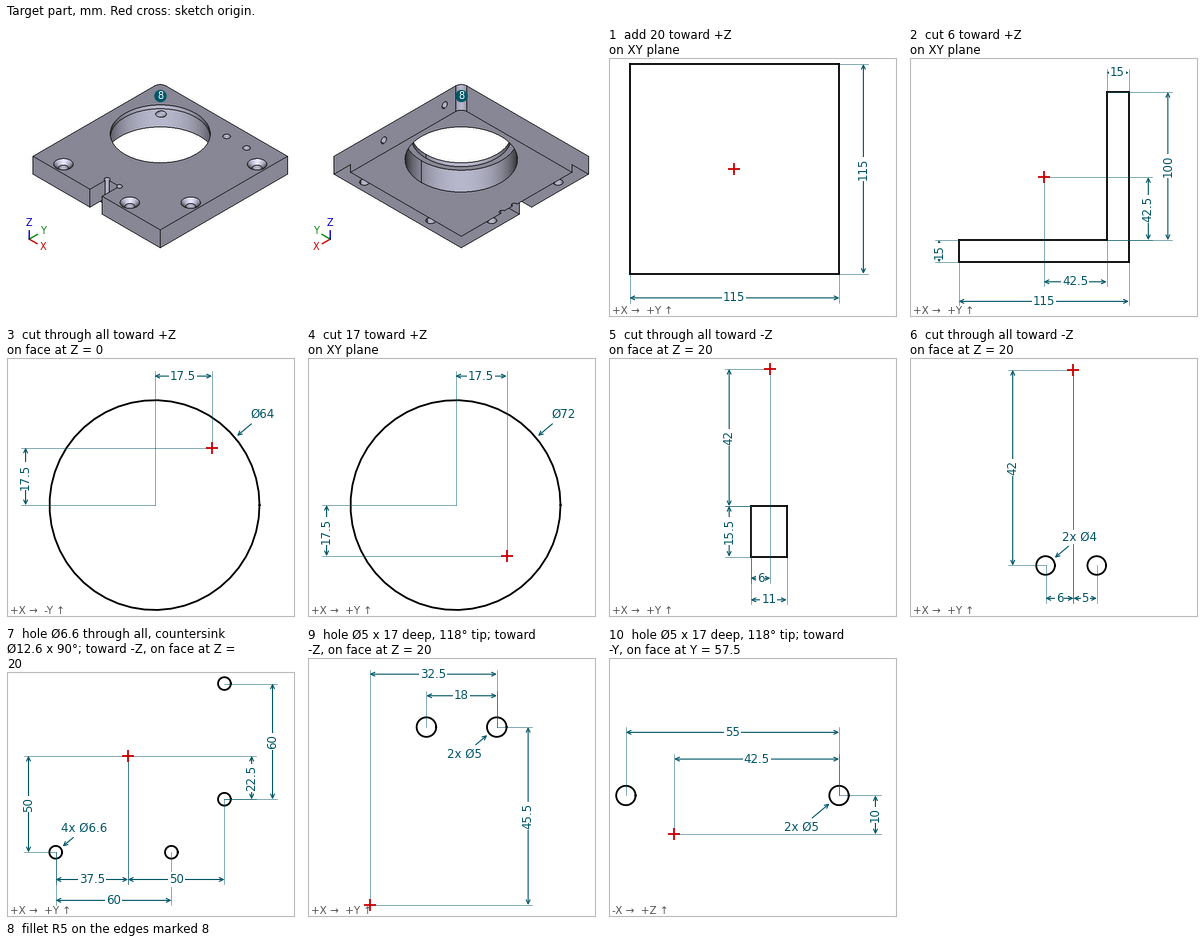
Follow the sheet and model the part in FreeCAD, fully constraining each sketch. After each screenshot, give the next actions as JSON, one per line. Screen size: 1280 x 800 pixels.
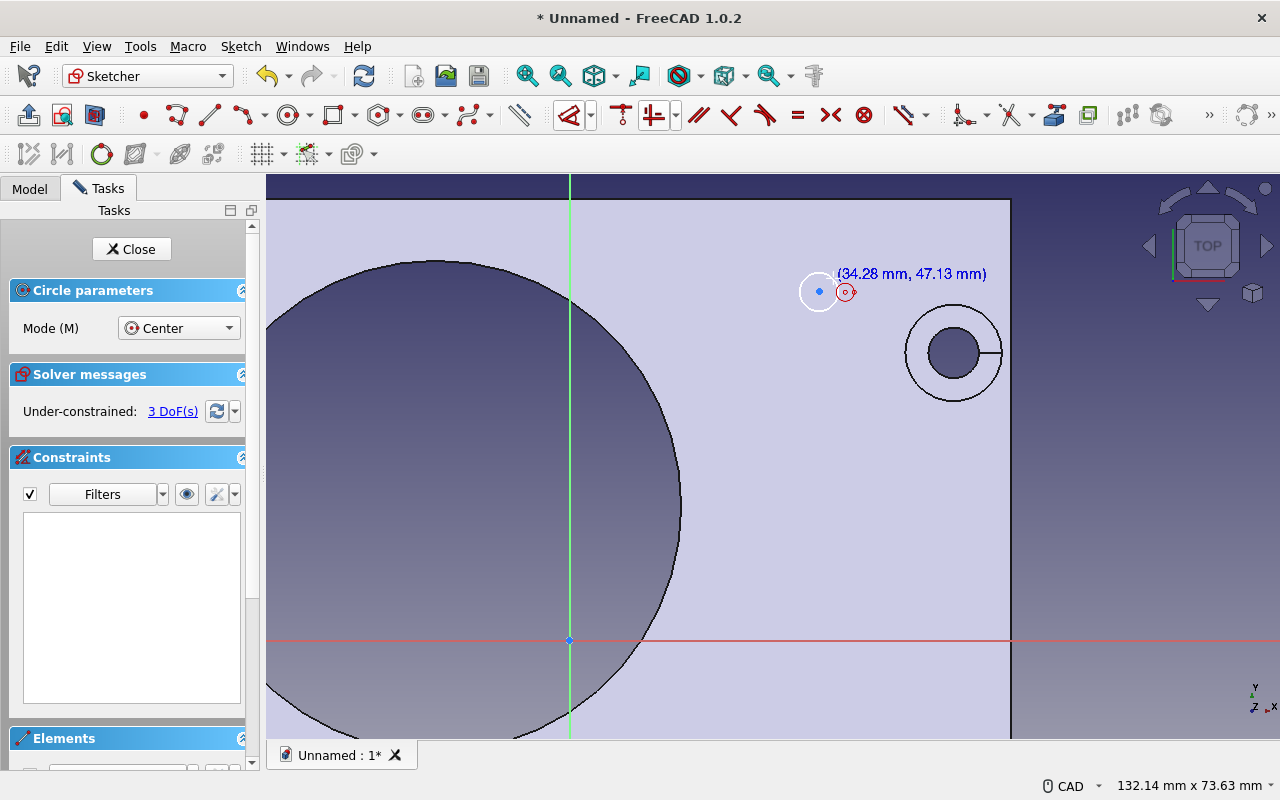
{"action": "left_click", "coordinate": [681, 291]}
{"action": "left_click", "coordinate": [695, 278]}
{"action": "key", "text": "Escape"}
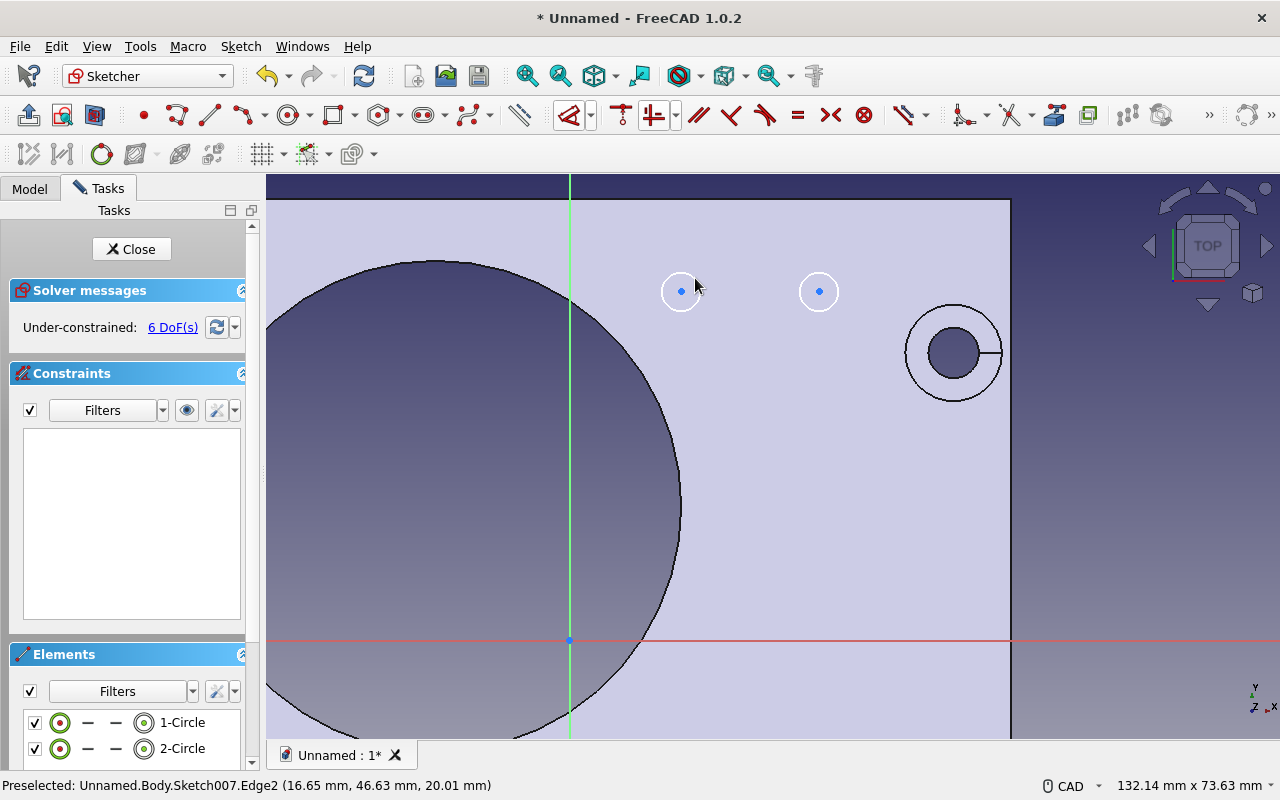
{"action": "left_click", "coordinate": [832, 278]}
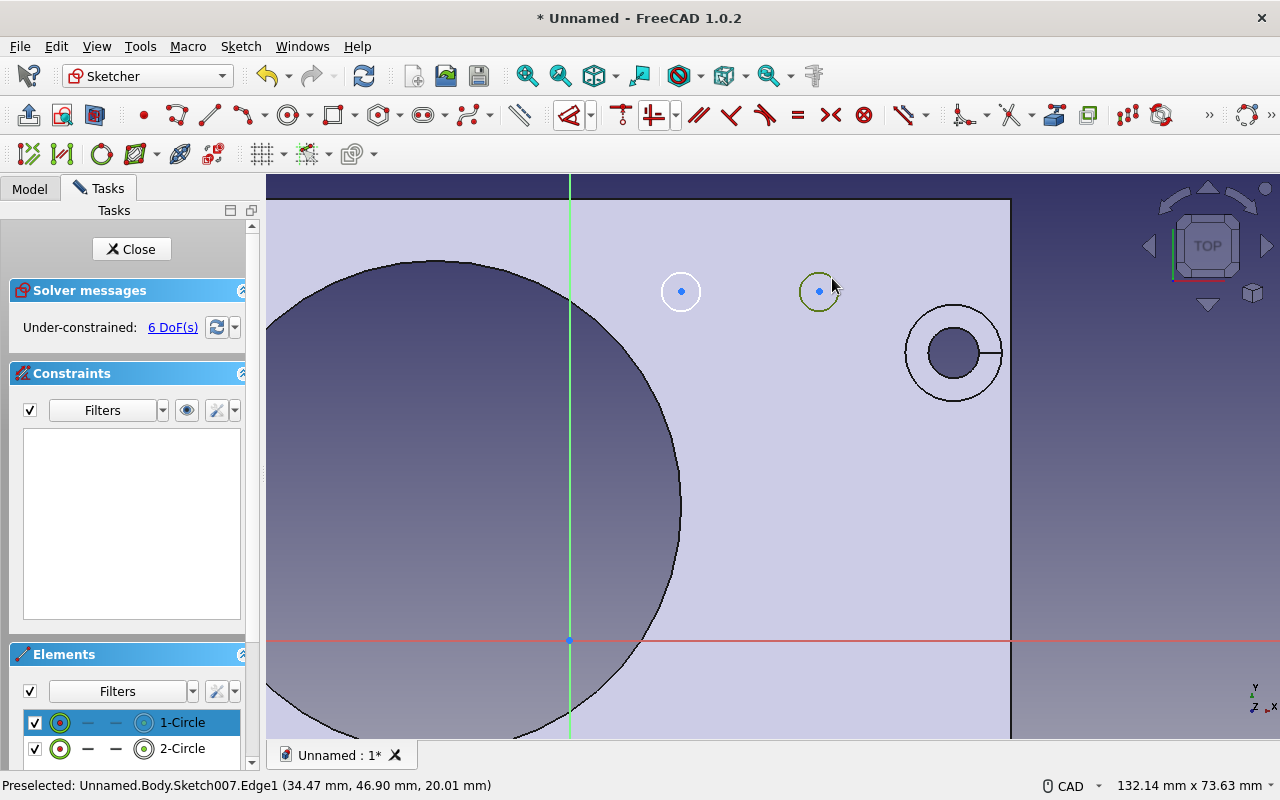
{"action": "left_click", "coordinate": [694, 278]}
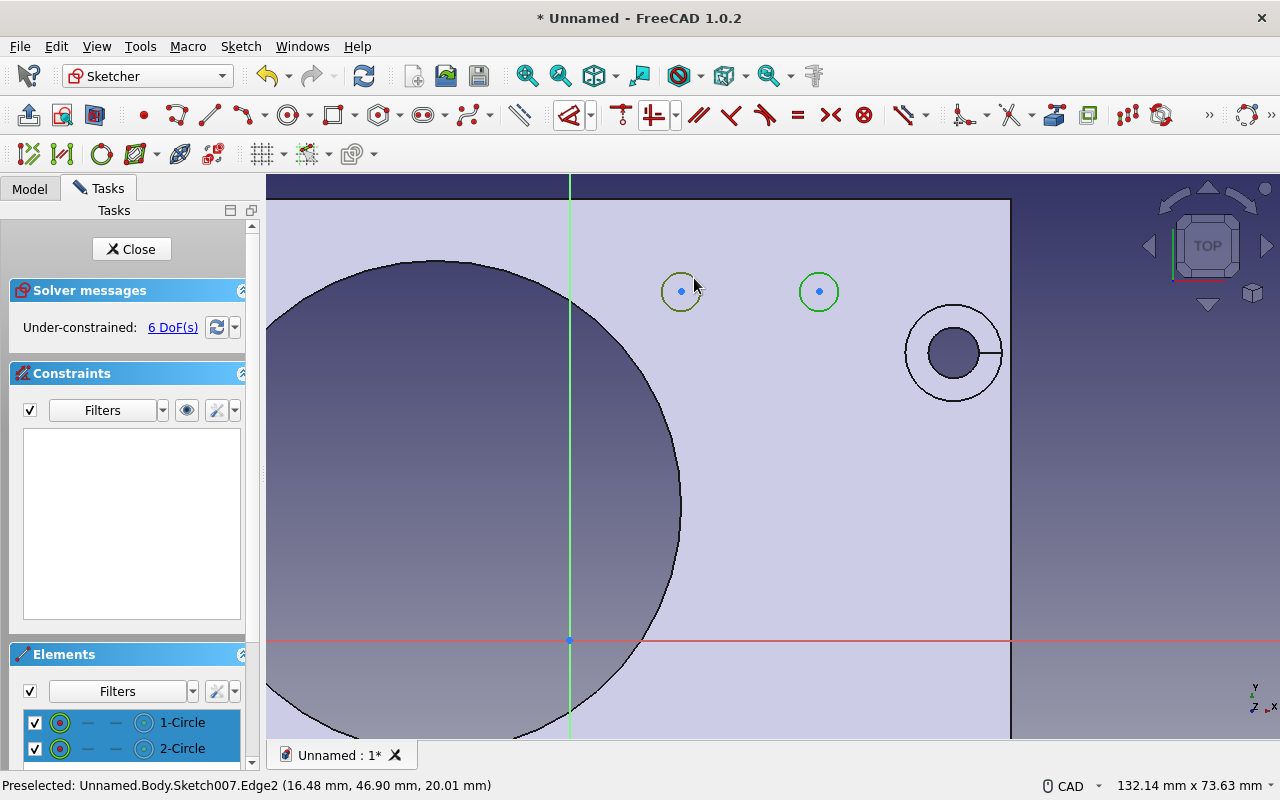
{"action": "left_click", "coordinate": [798, 116]}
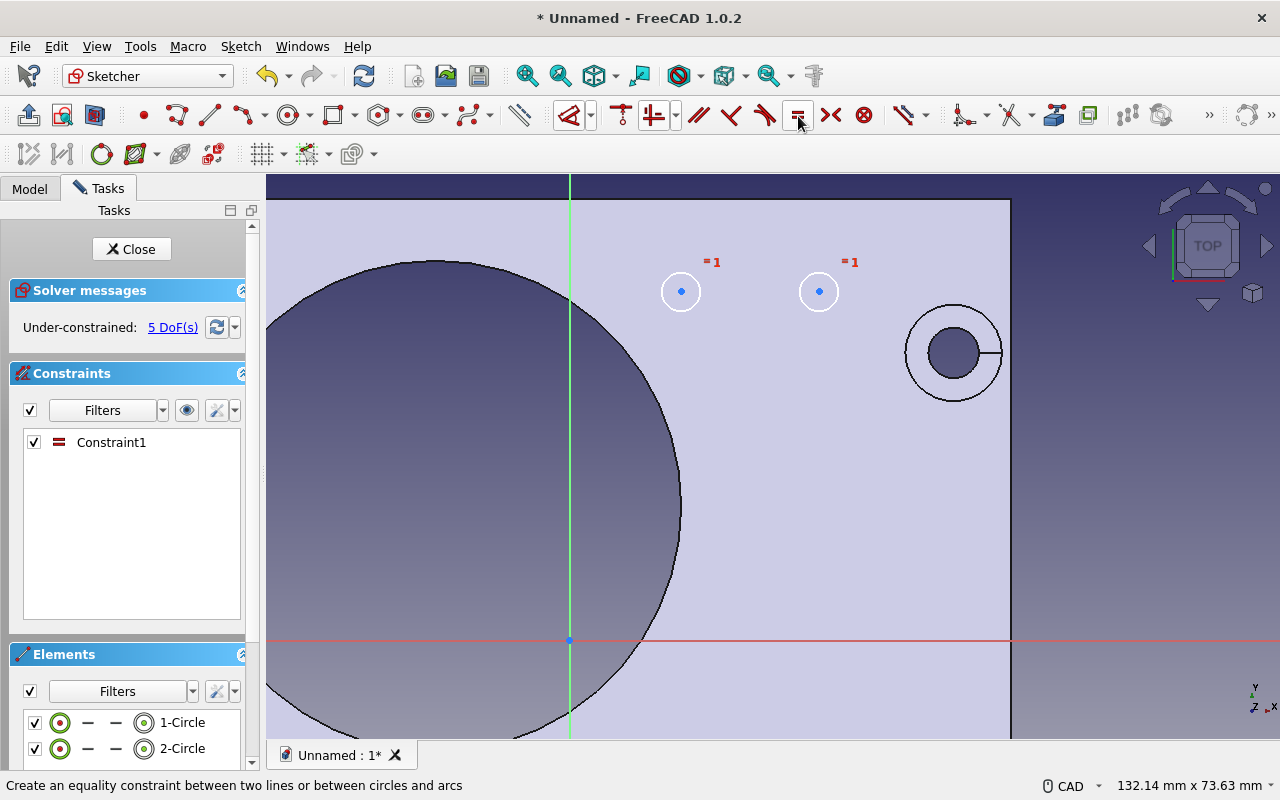
{"action": "left_click", "coordinate": [819, 292]}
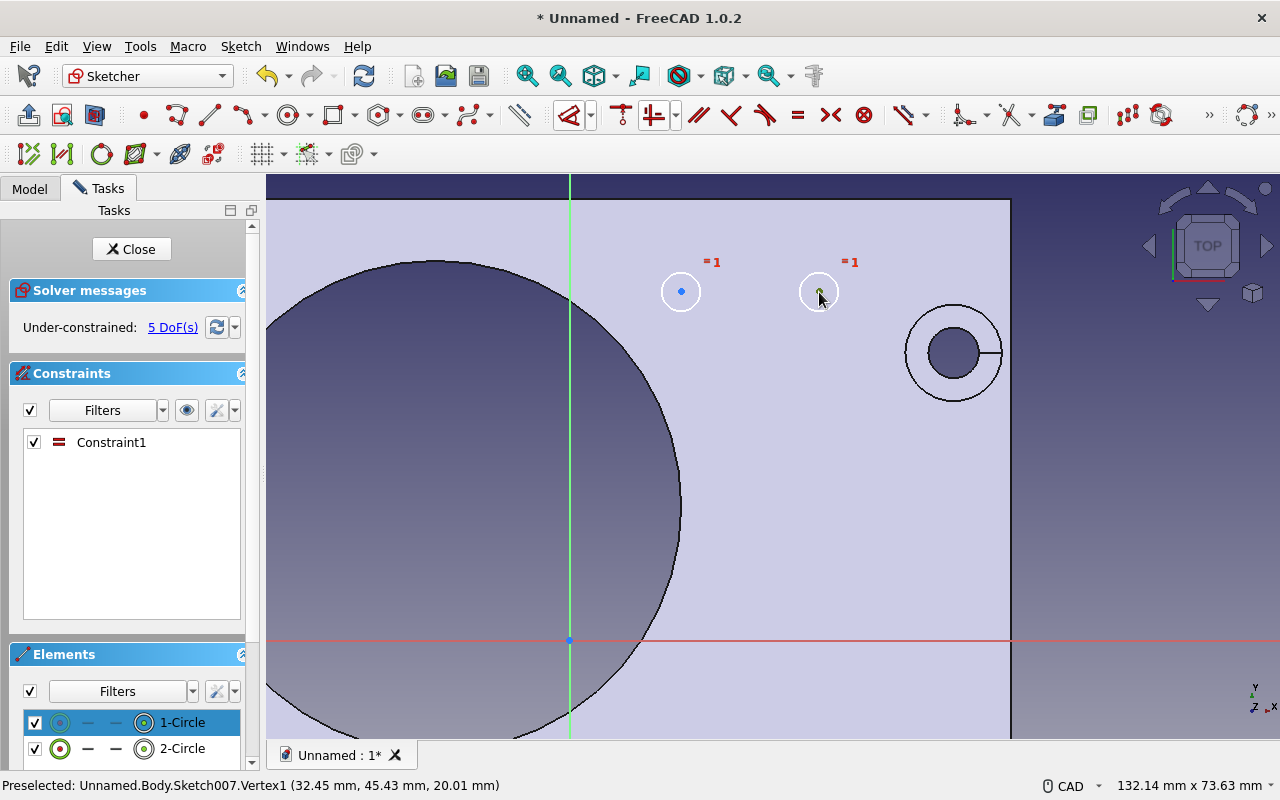
{"action": "left_click", "coordinate": [681, 292]}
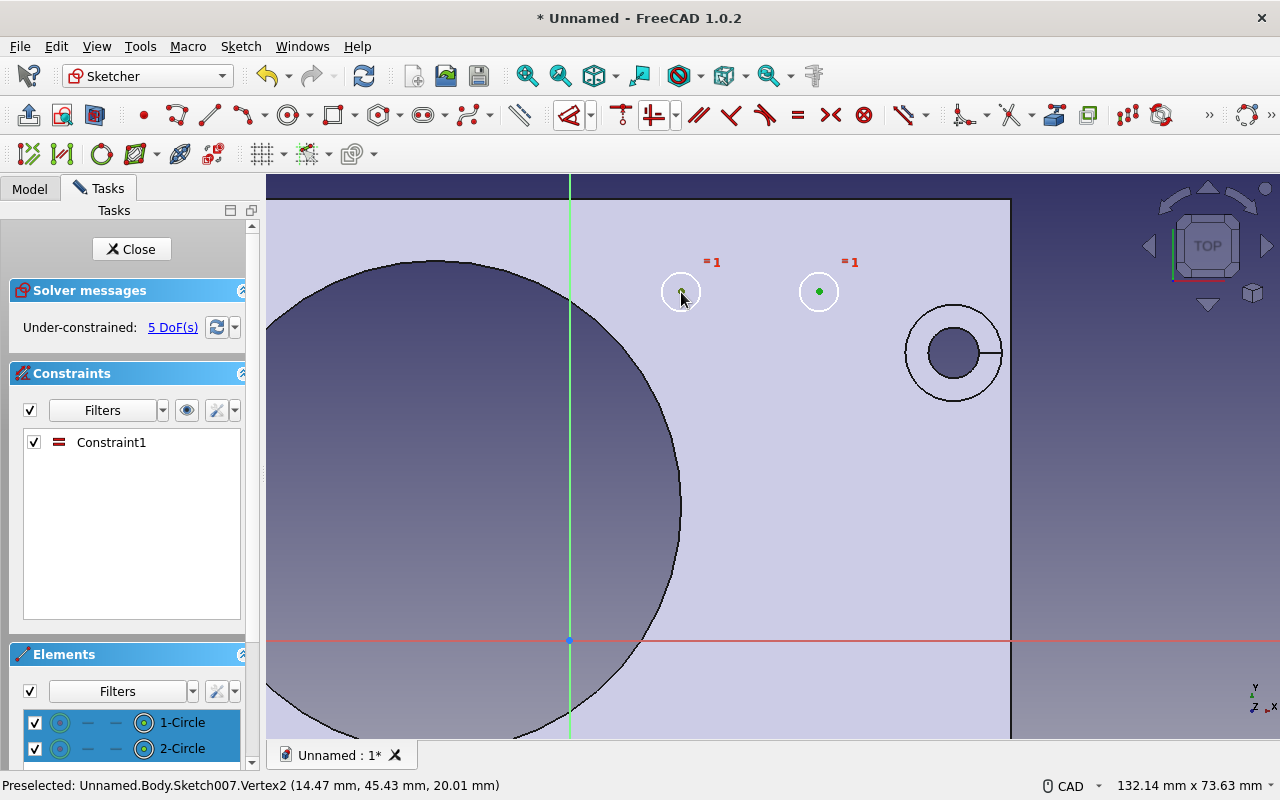
{"action": "key", "text": "h"}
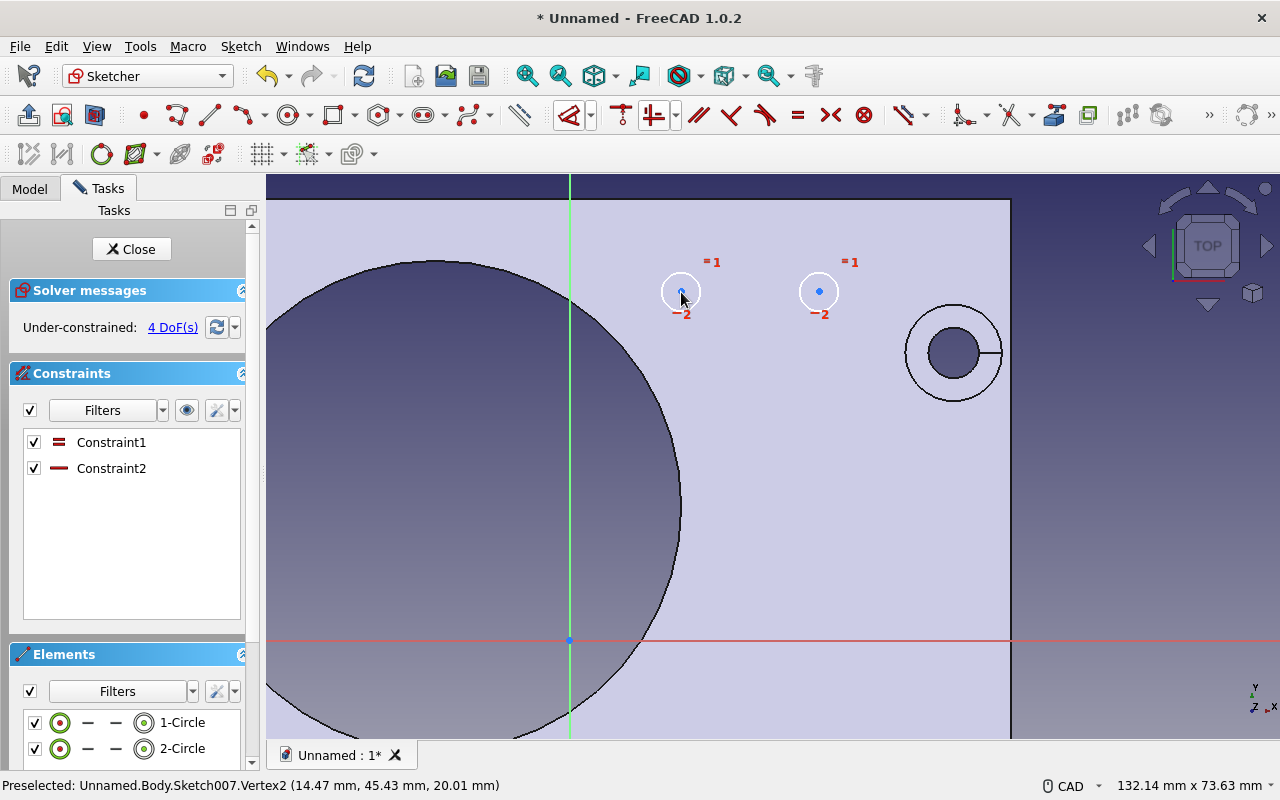
{"action": "left_click", "coordinate": [832, 278]}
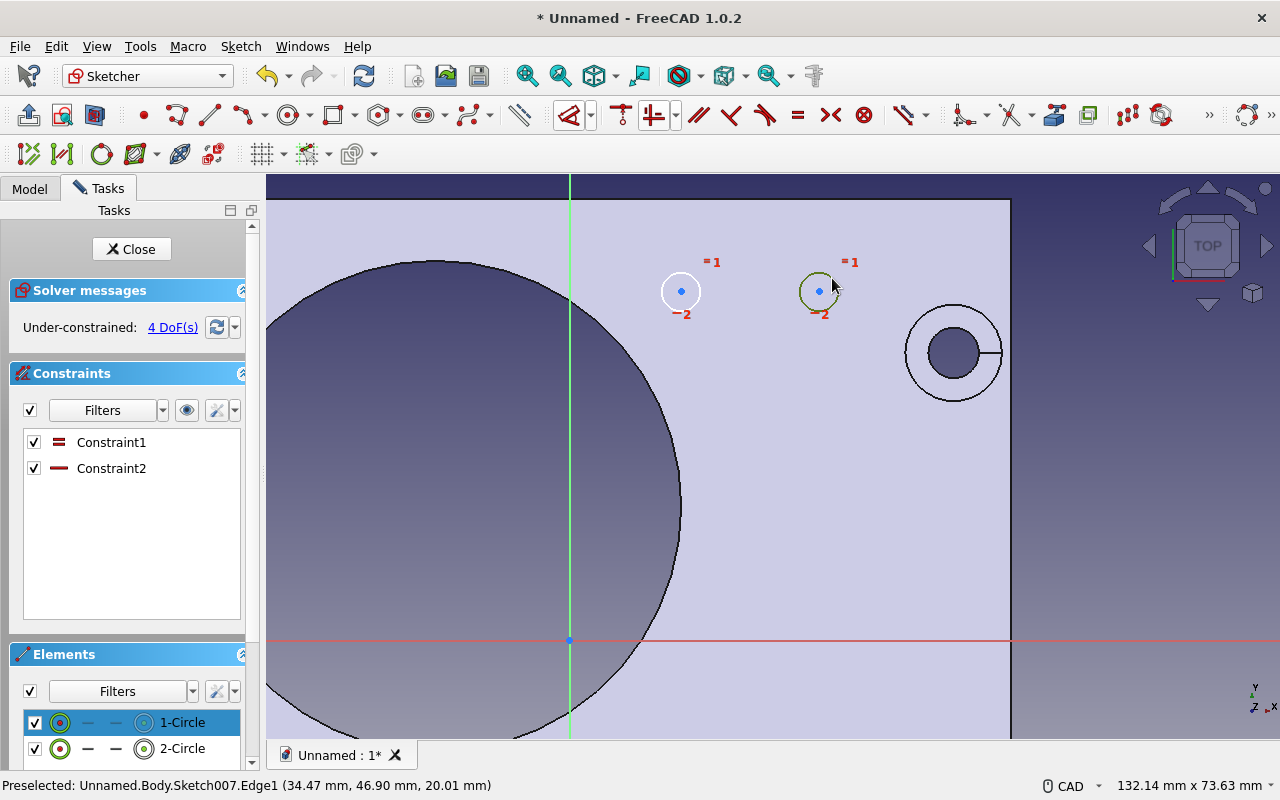
{"action": "key", "text": "k o"}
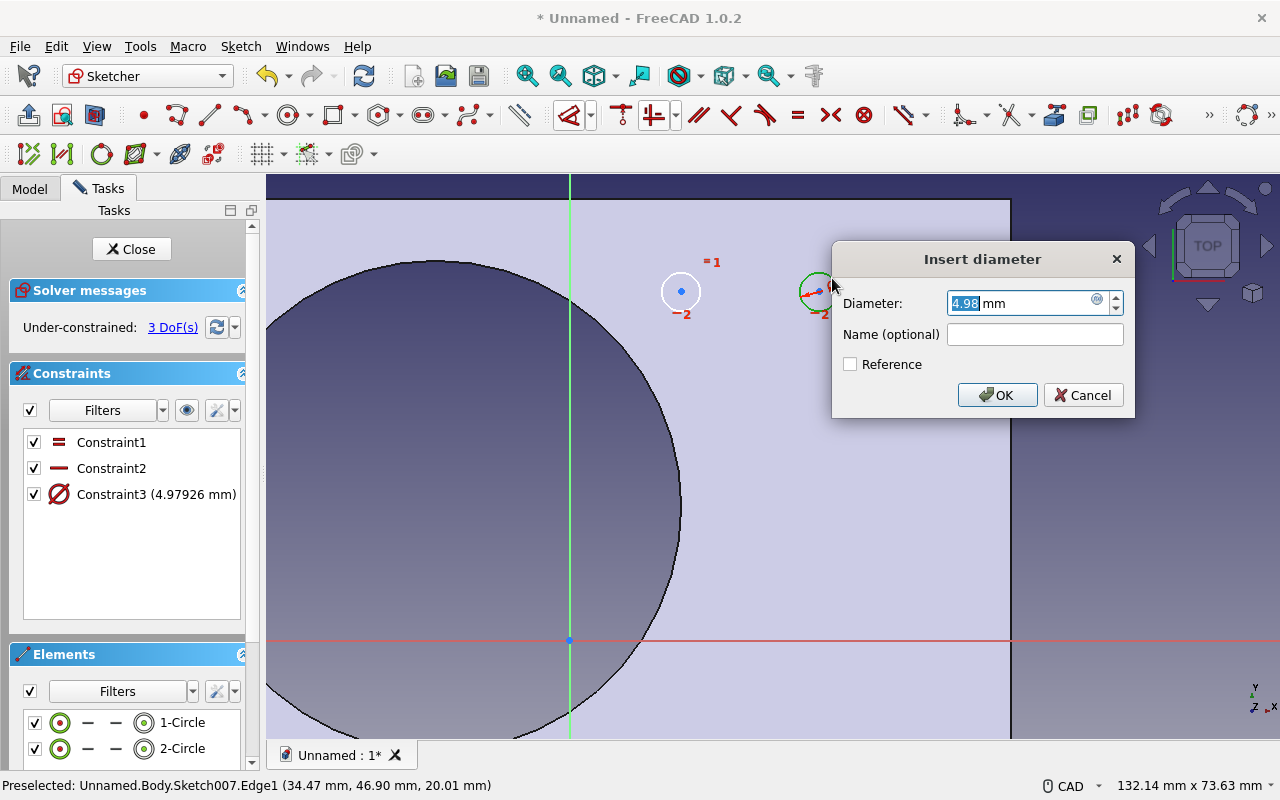
{"action": "type", "text": "5"}
{"action": "key", "text": "Return"}